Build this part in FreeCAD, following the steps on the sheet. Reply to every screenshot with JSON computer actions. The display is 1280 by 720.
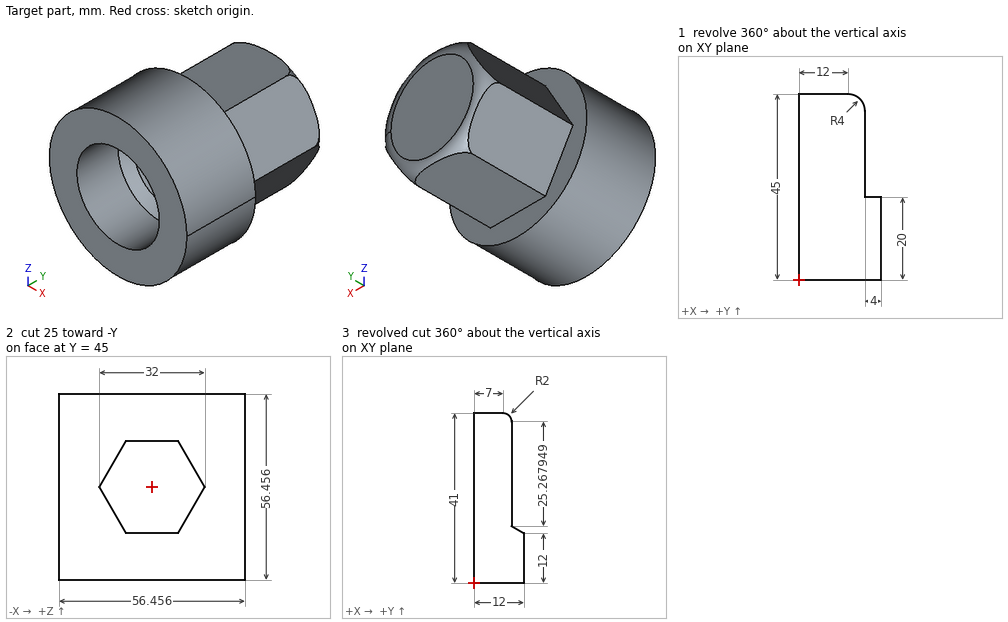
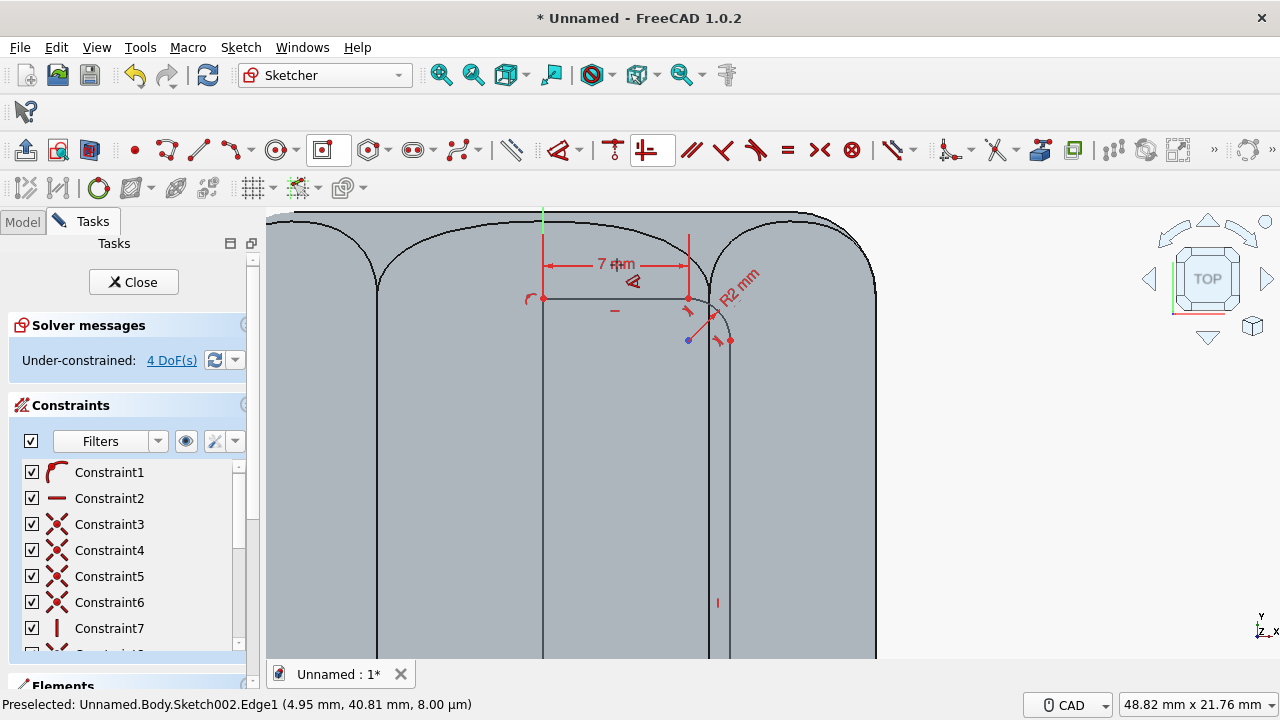
{"action": "left_click", "coordinate": [543, 553]}
{"action": "left_click", "coordinate": [509, 465]}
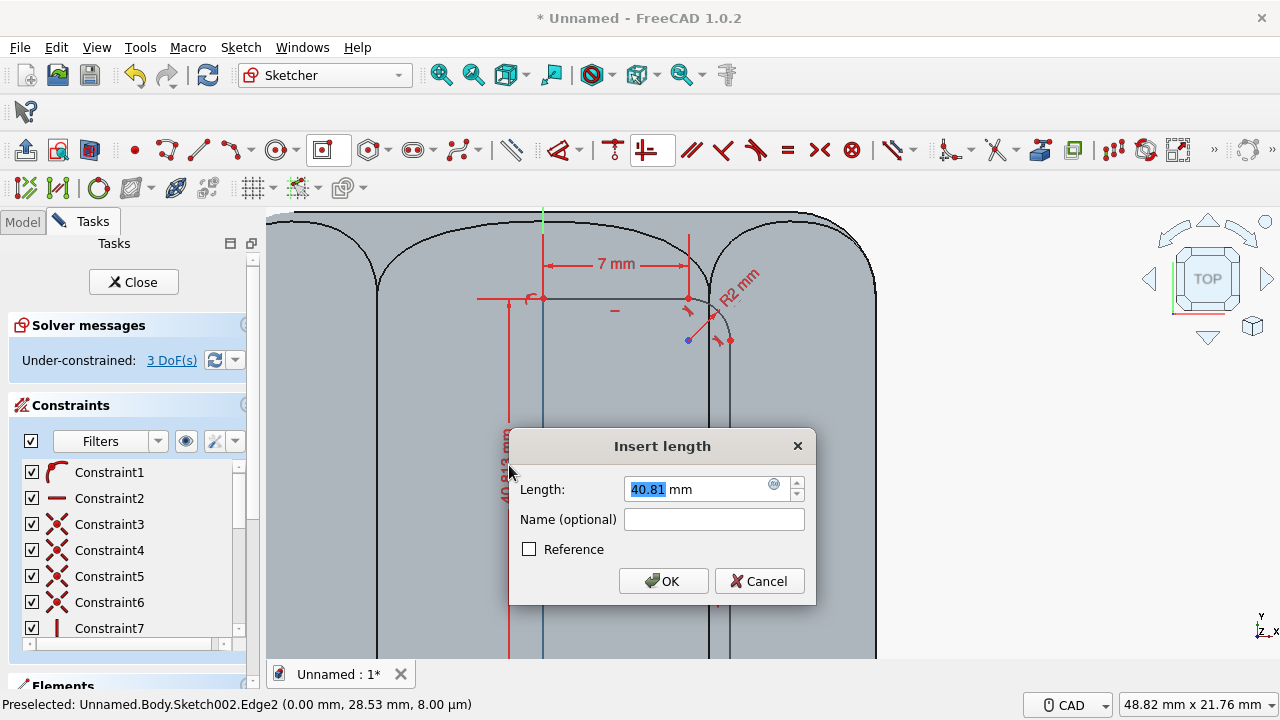
{"action": "type", "text": "41"}
{"action": "key", "text": "Return"}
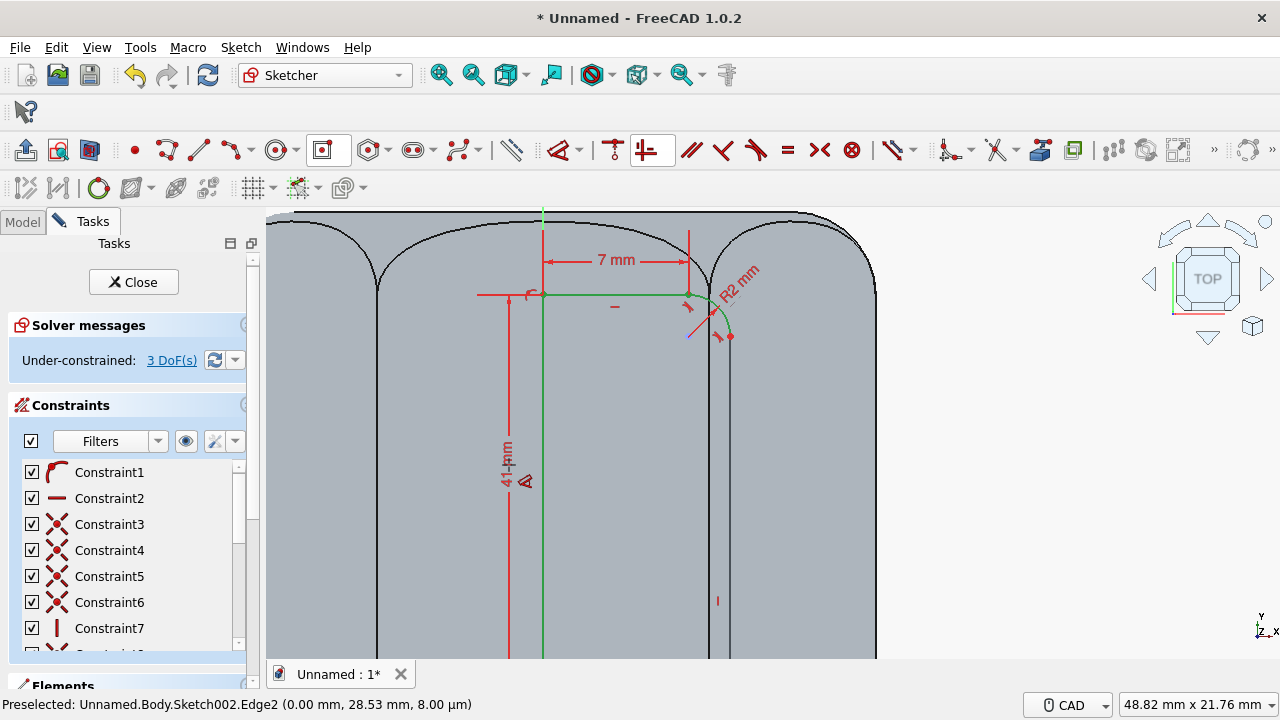
{"action": "scroll", "coordinate": [720, 309], "scroll_direction": "down", "scroll_amount": 6}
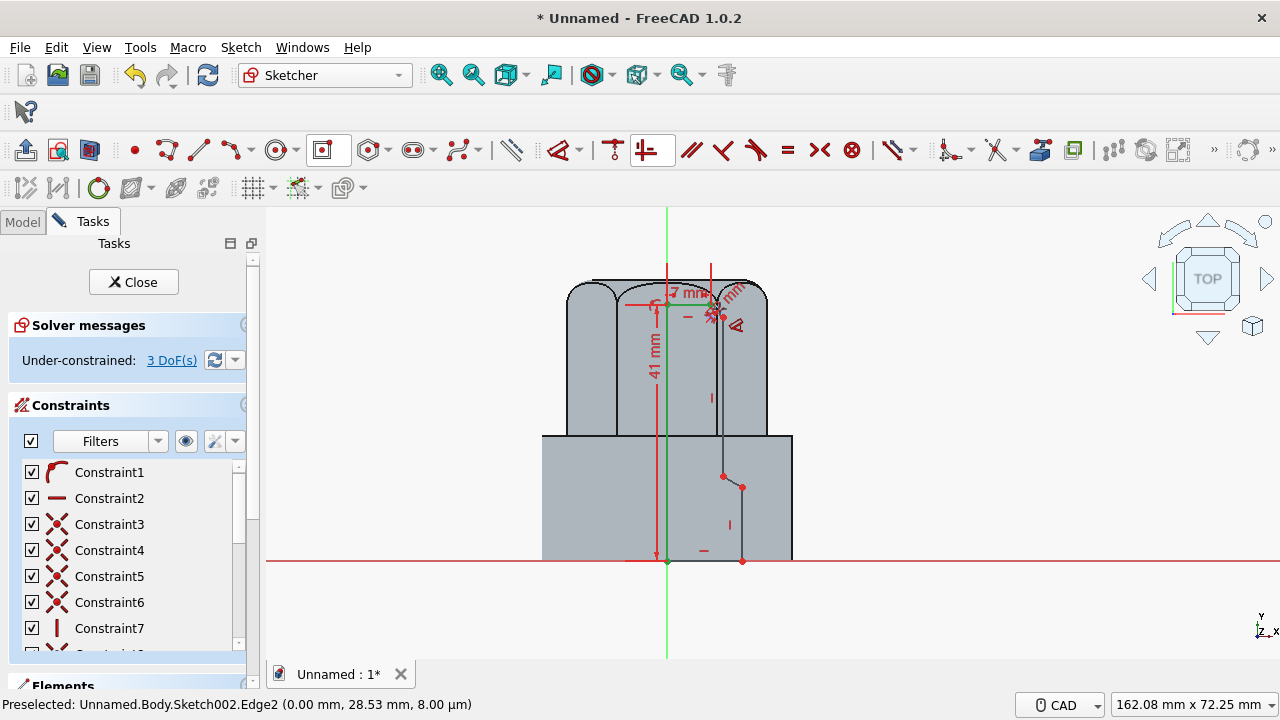
{"action": "left_click", "coordinate": [690, 561]}
{"action": "left_click", "coordinate": [705, 595]}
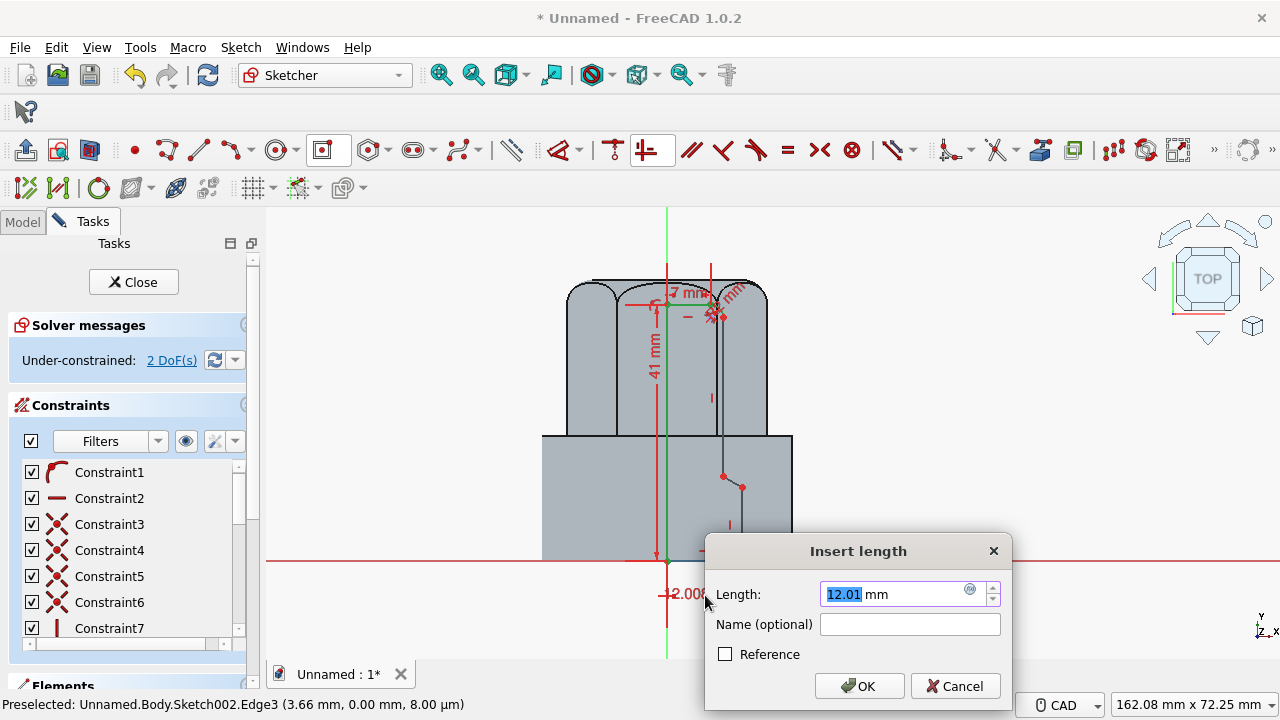
{"action": "type", "text": "12"}
{"action": "key", "text": "Return"}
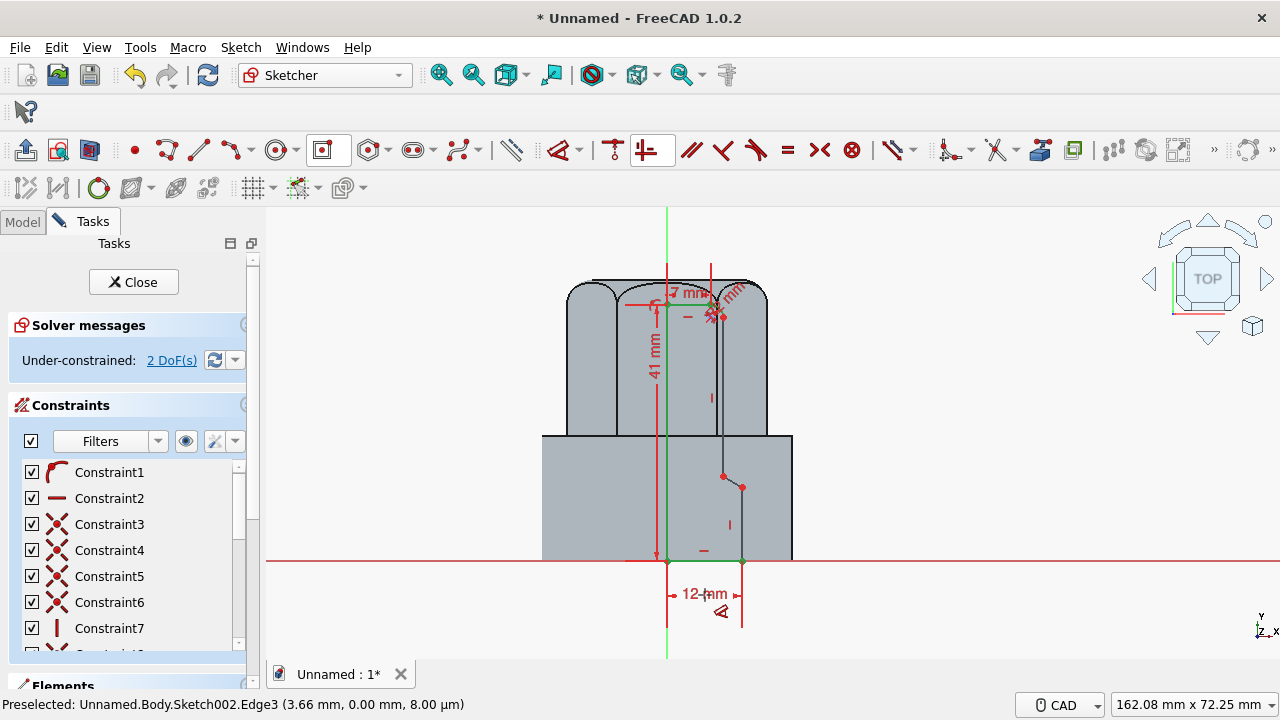
{"action": "left_click", "coordinate": [742, 539]}
{"action": "left_click", "coordinate": [776, 525]}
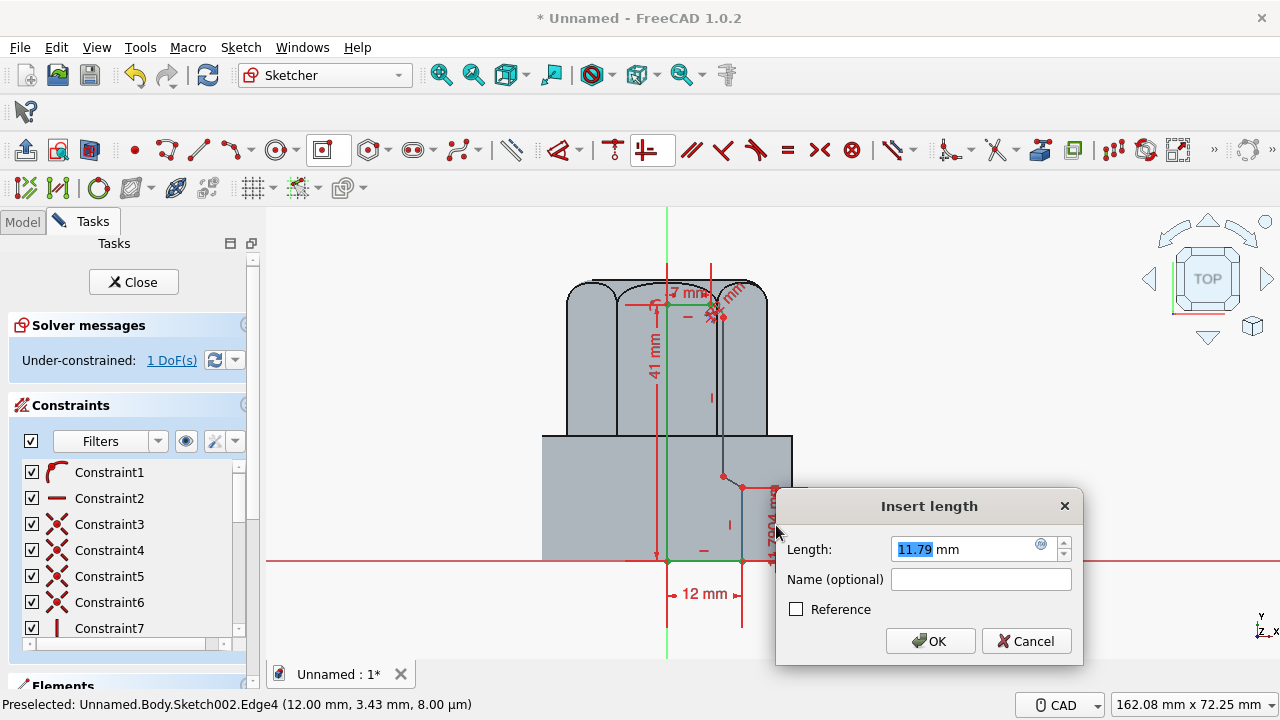
{"action": "type", "text": "12"}
{"action": "key", "text": "Return"}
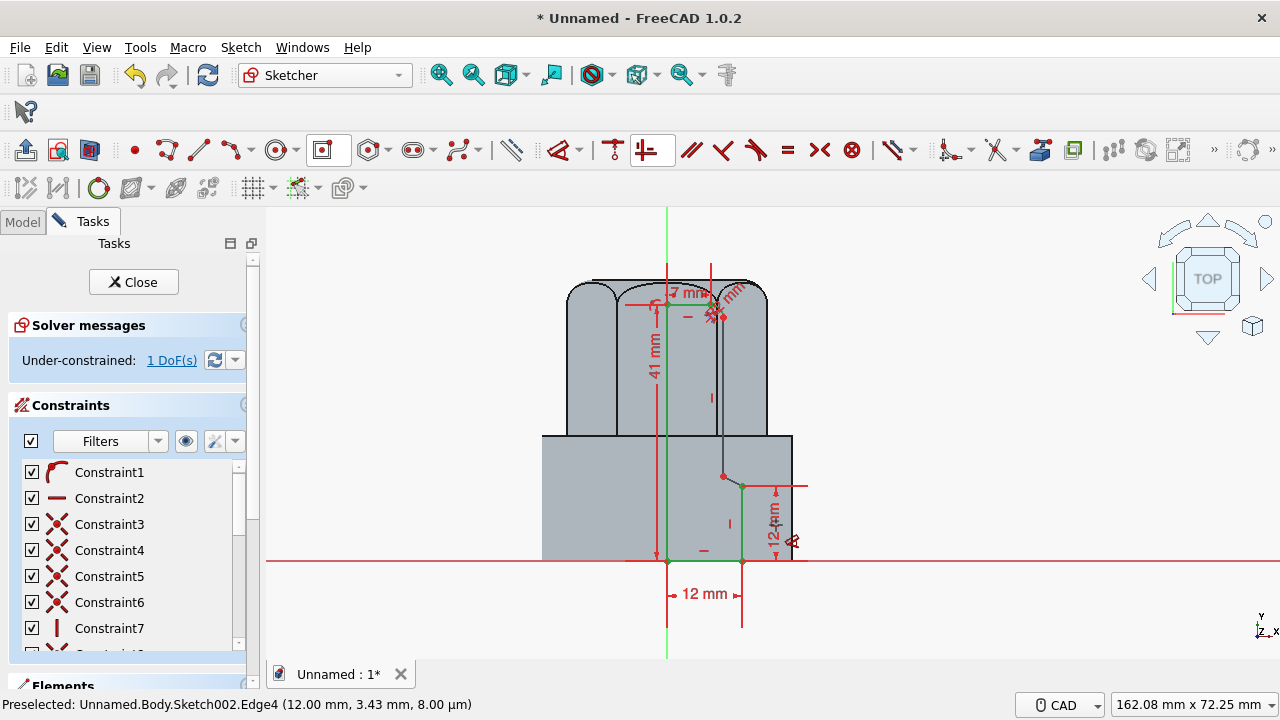
{"action": "left_click", "coordinate": [723, 429]}
{"action": "left_click", "coordinate": [757, 397]}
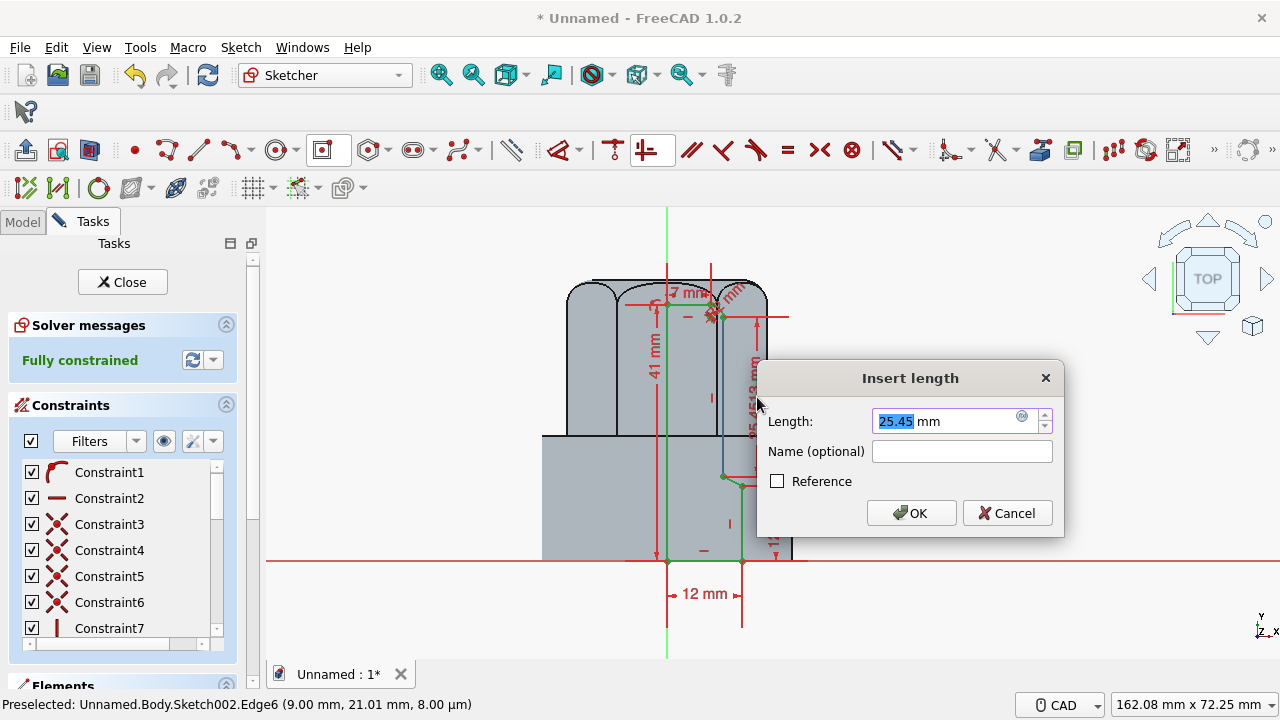
{"action": "type", "text": "25.267949"}
{"action": "key", "text": "Return"}
{"action": "key", "text": "Escape"}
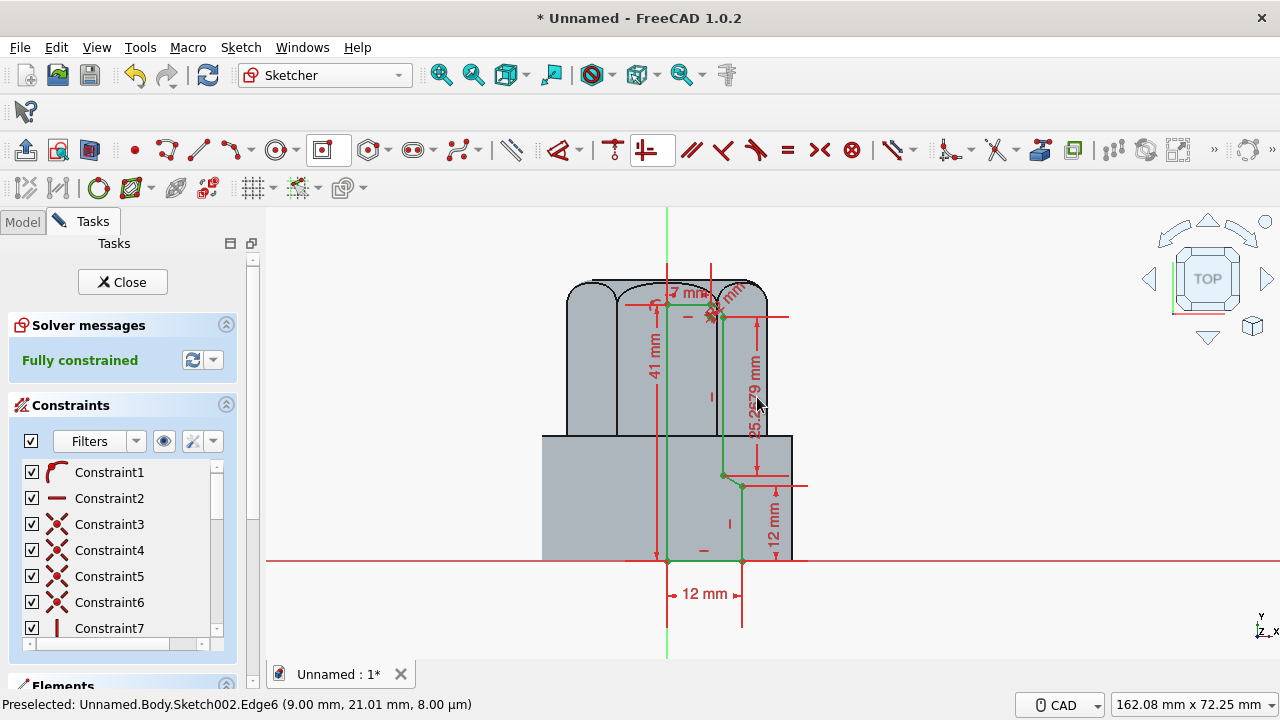
{"action": "left_click", "coordinate": [123, 282]}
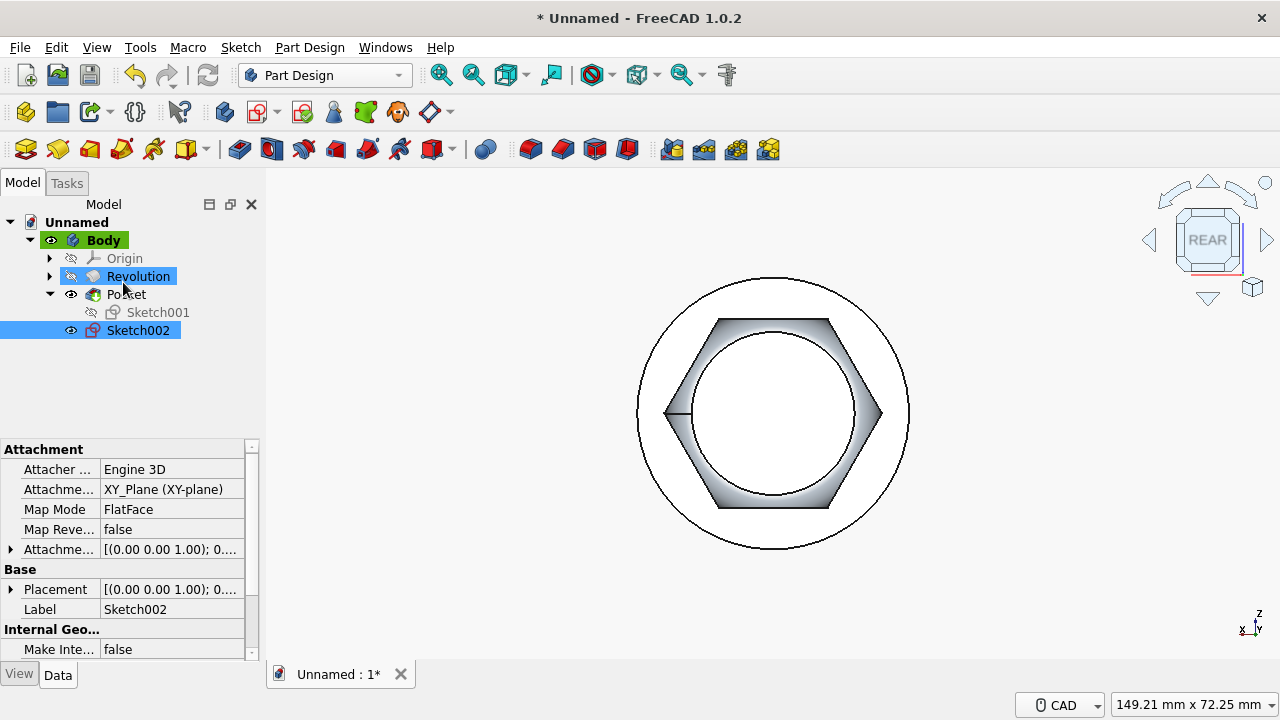
{"action": "left_click", "coordinate": [304, 150]}